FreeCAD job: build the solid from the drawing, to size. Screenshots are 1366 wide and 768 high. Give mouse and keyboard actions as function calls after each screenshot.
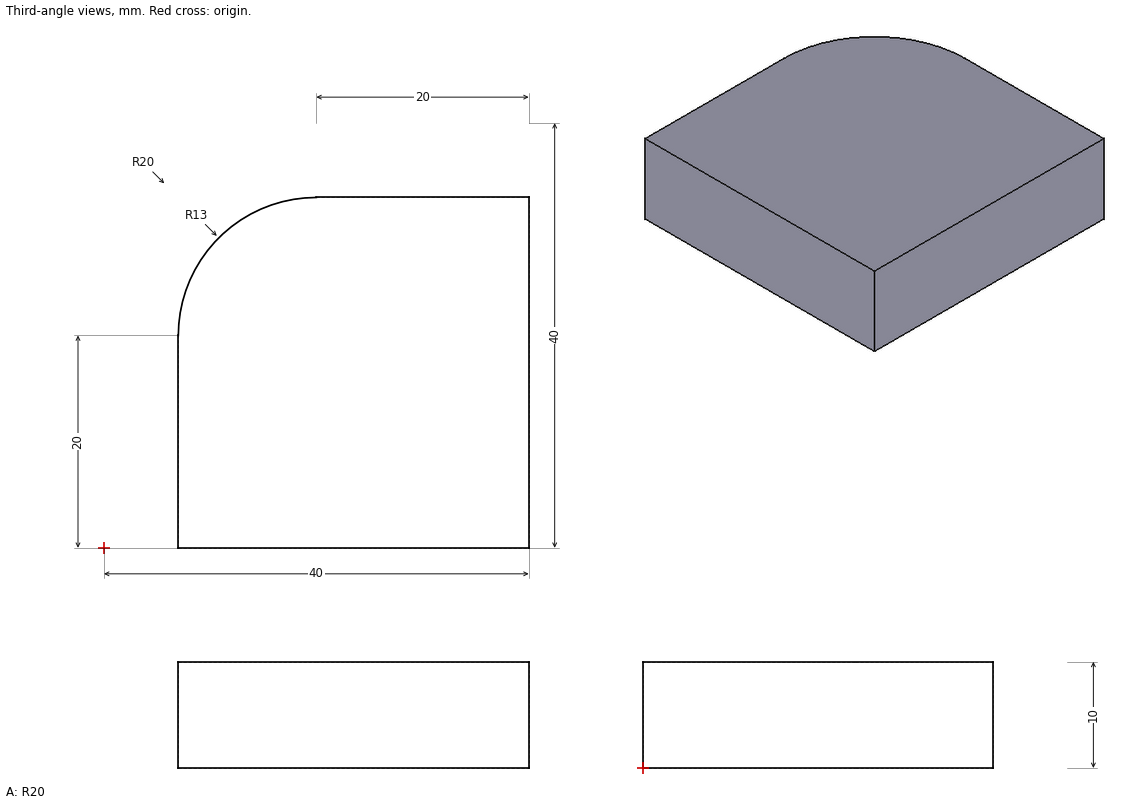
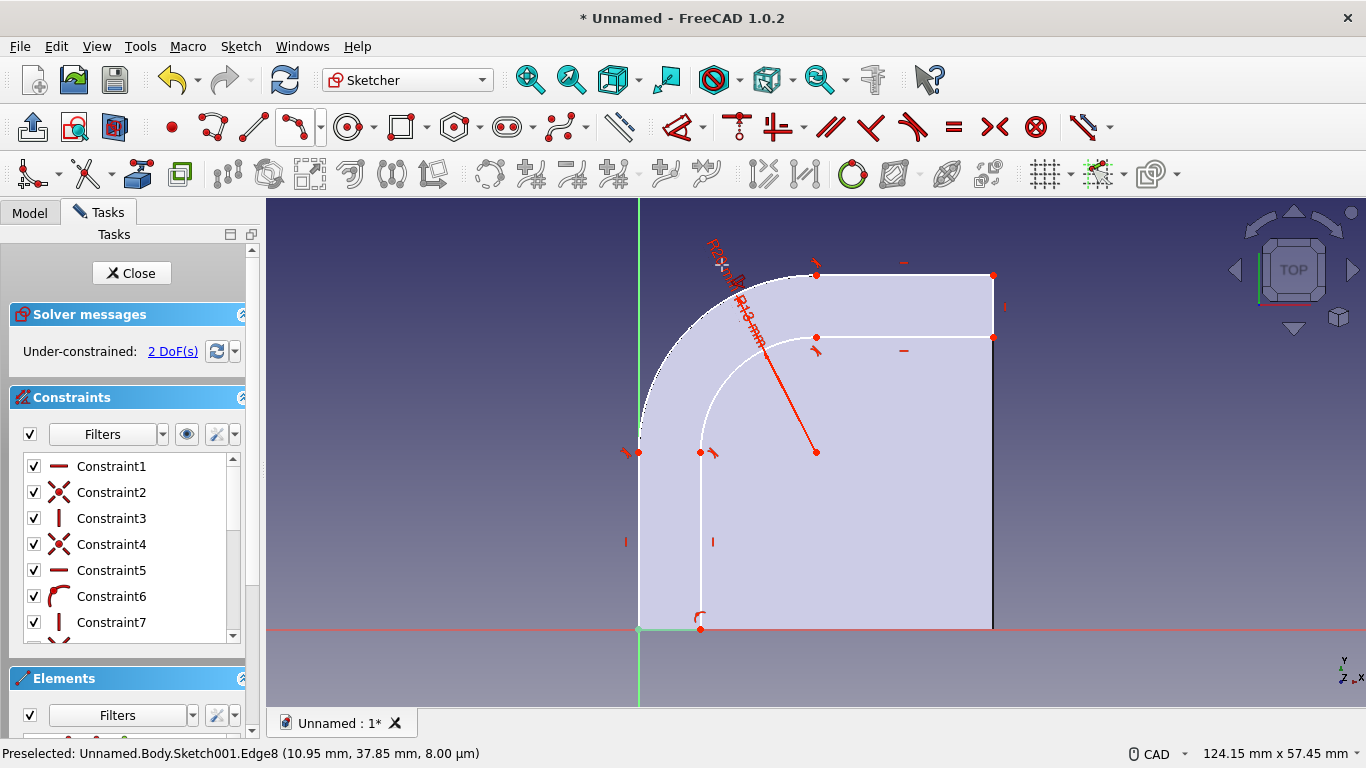
click(869, 275)
click(905, 241)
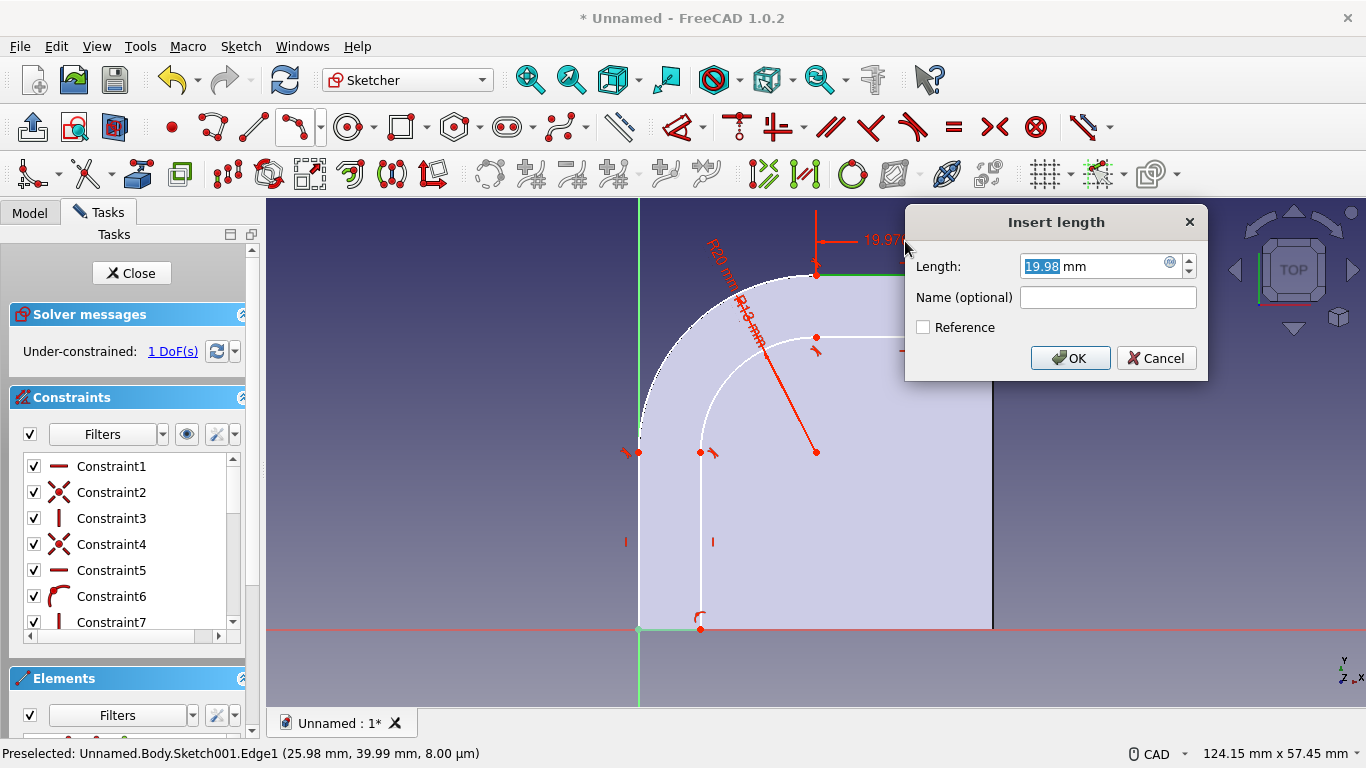
text(20)
key(Return)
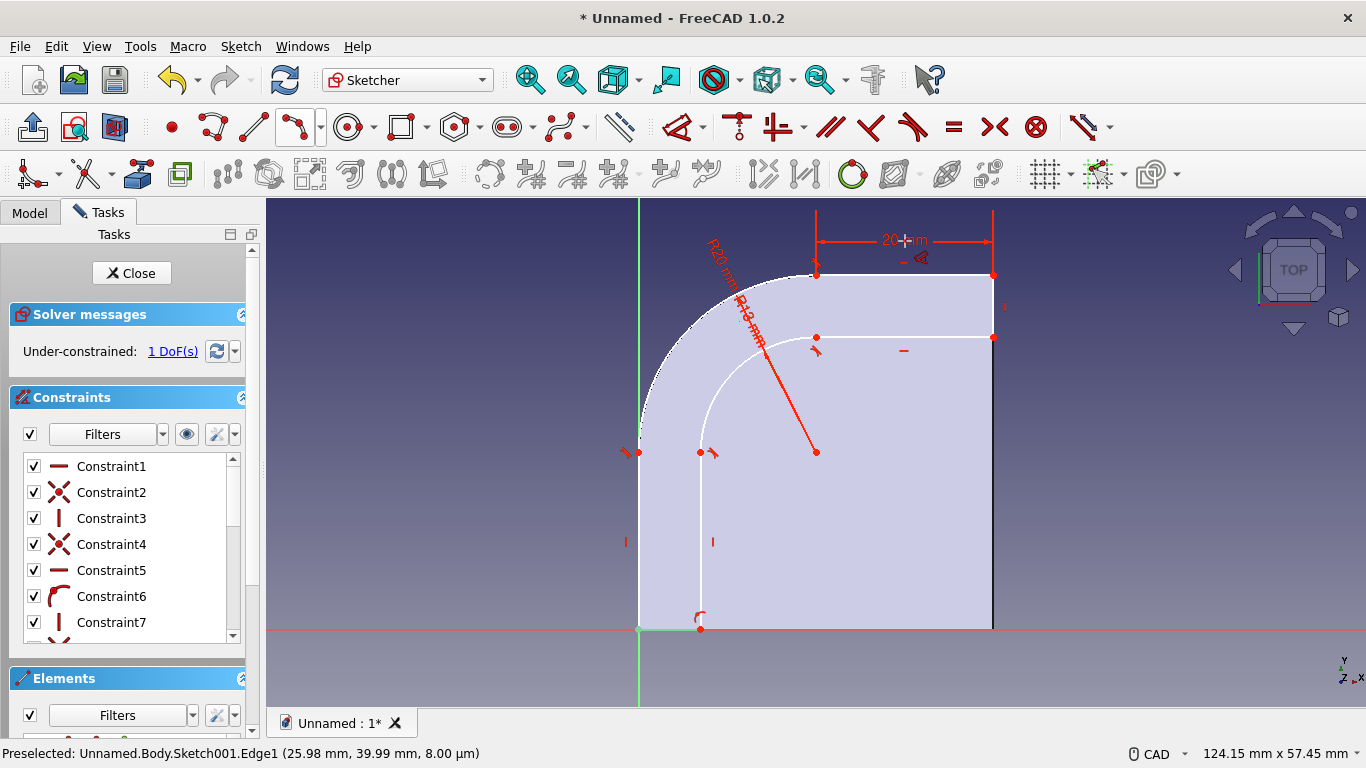
click(701, 506)
click(667, 541)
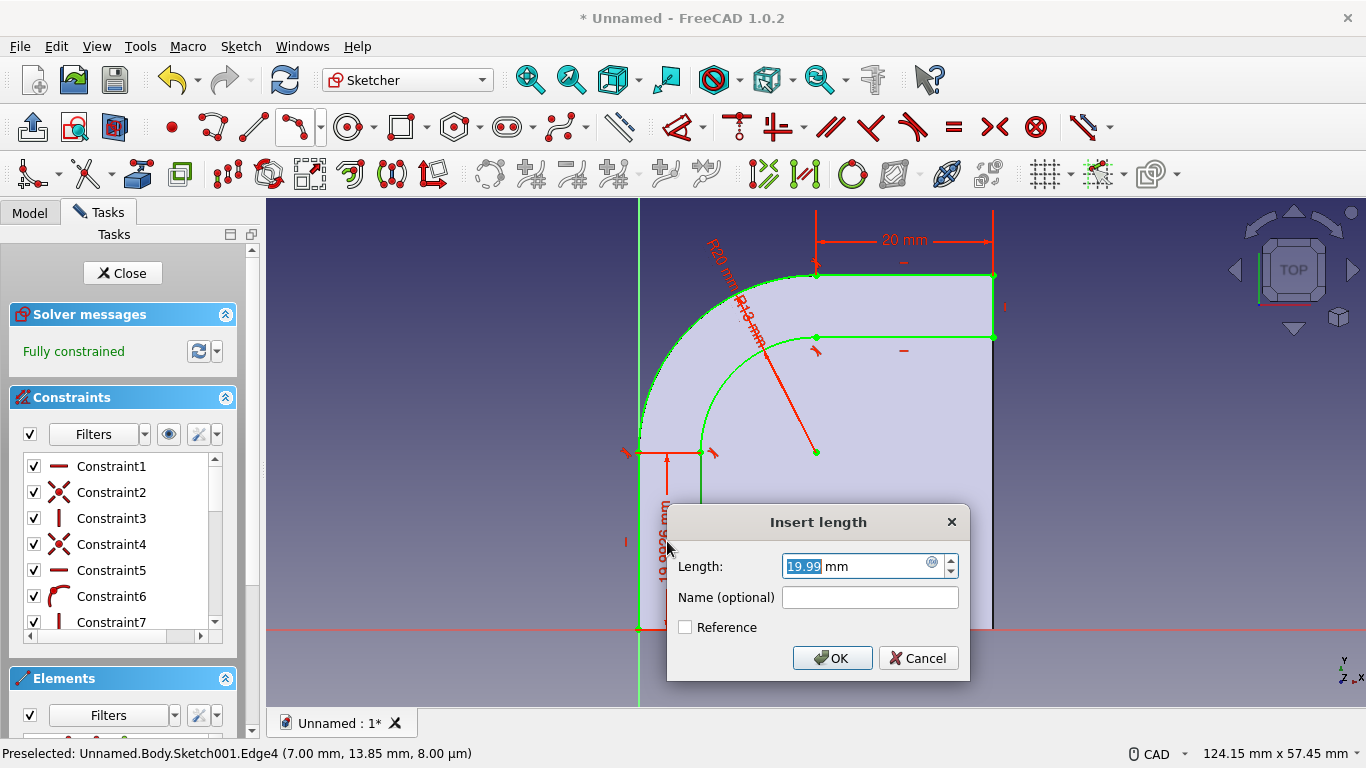
text(20)
key(Return)
key(Escape)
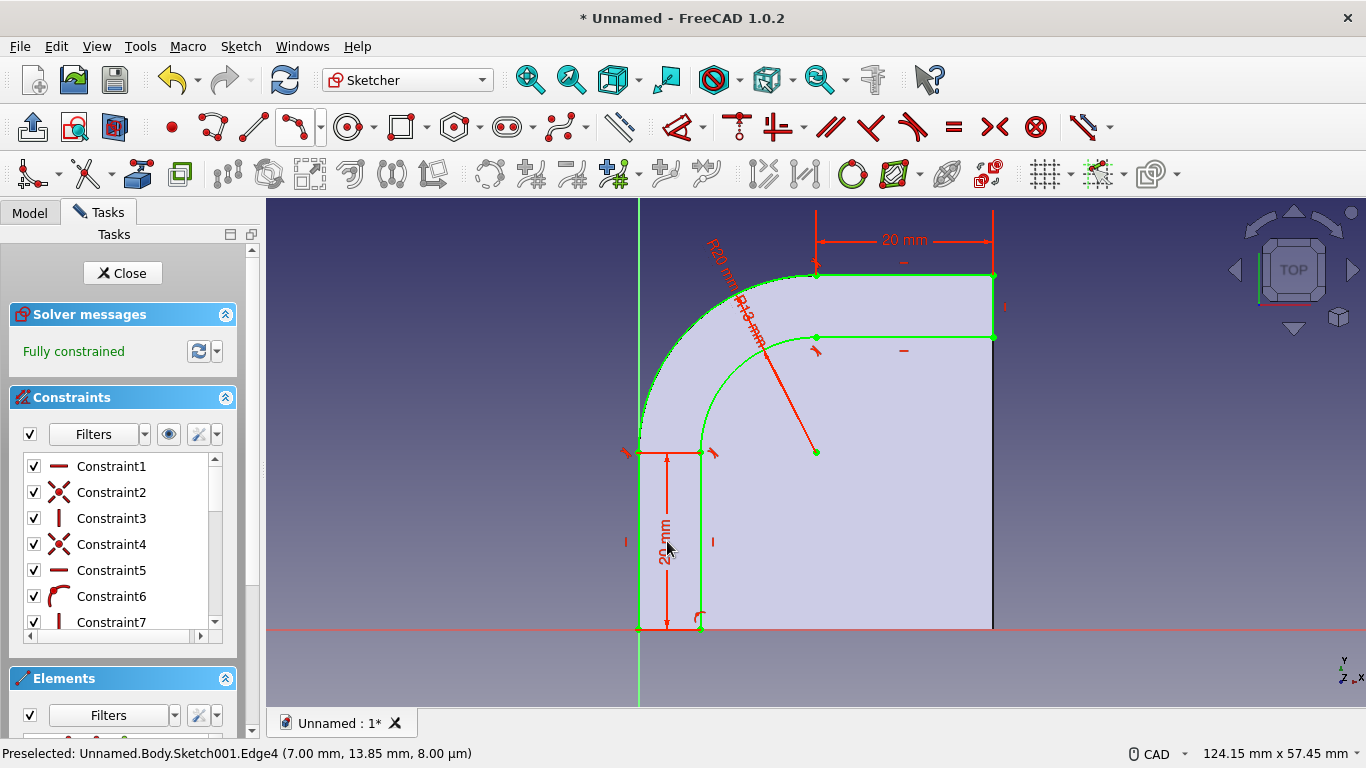
click(123, 273)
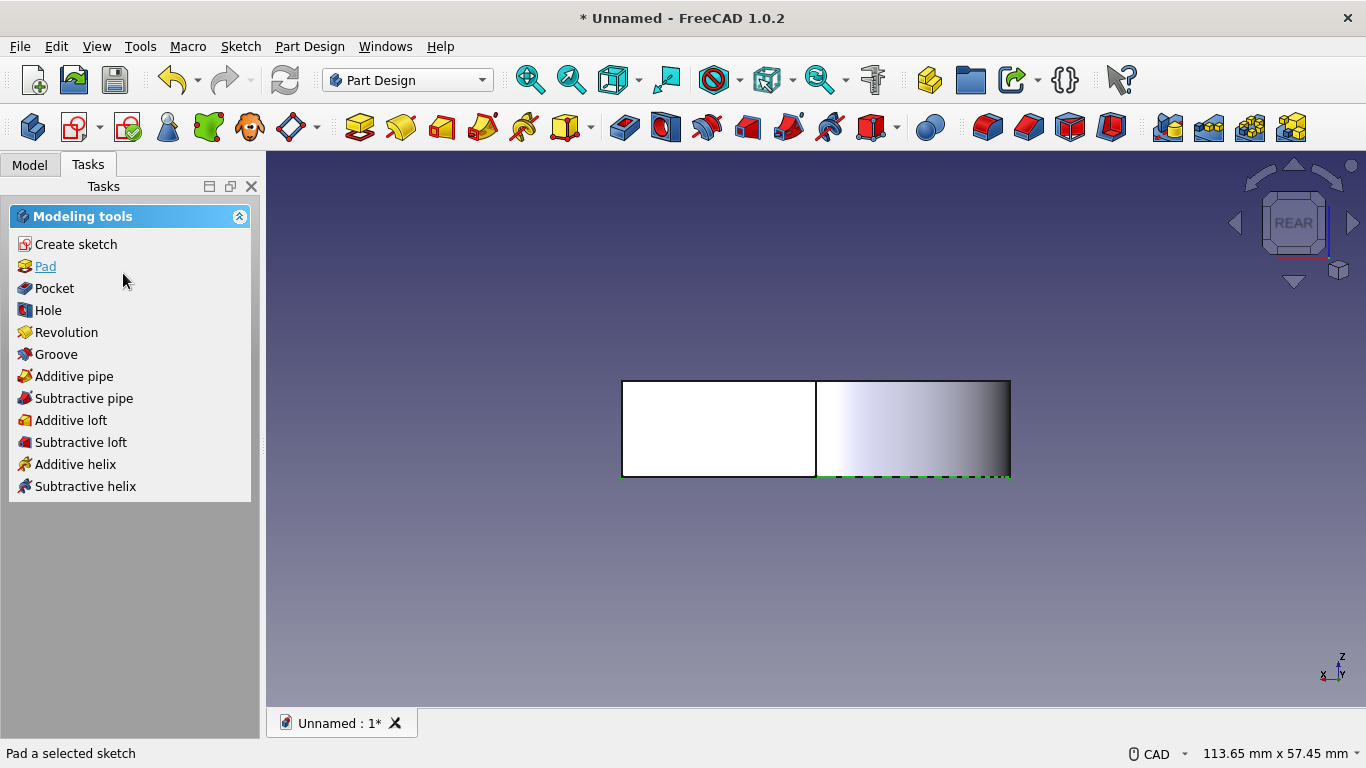
click(625, 128)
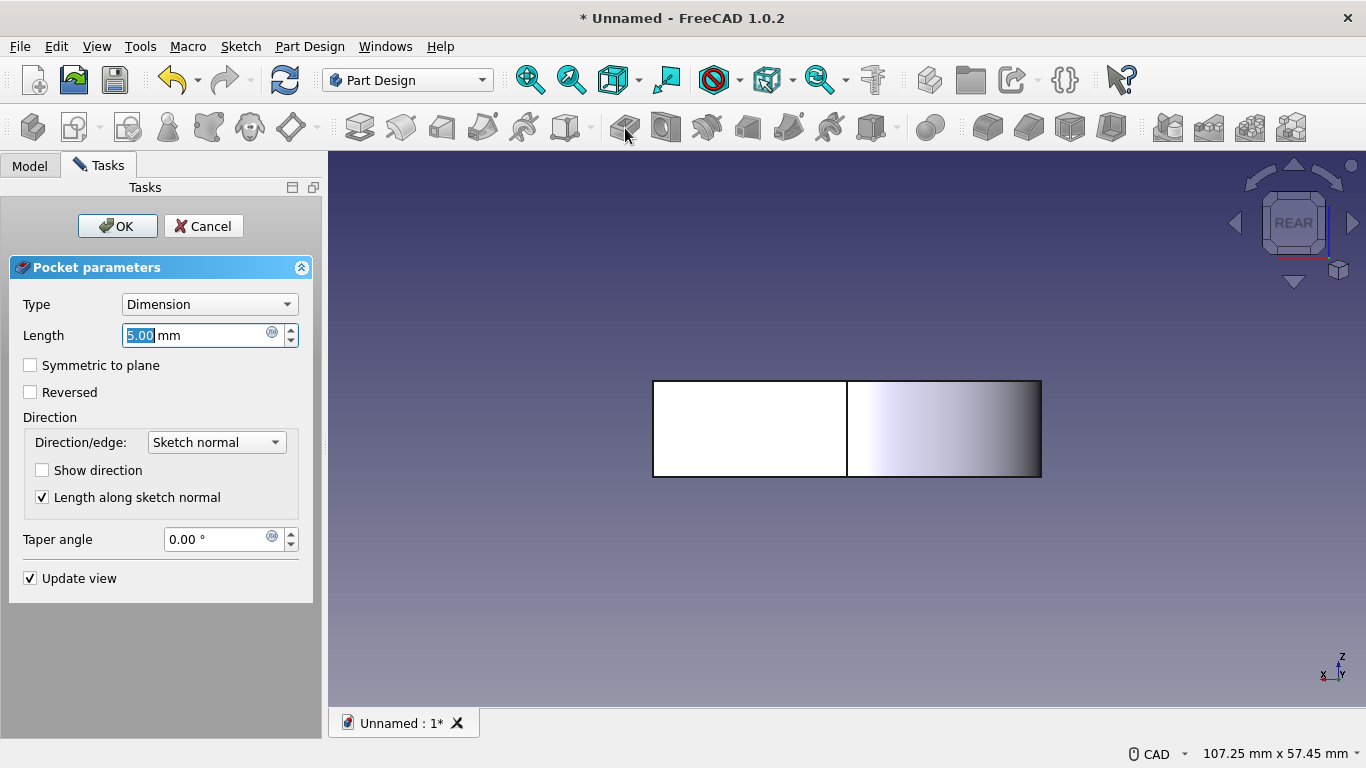
click(210, 304)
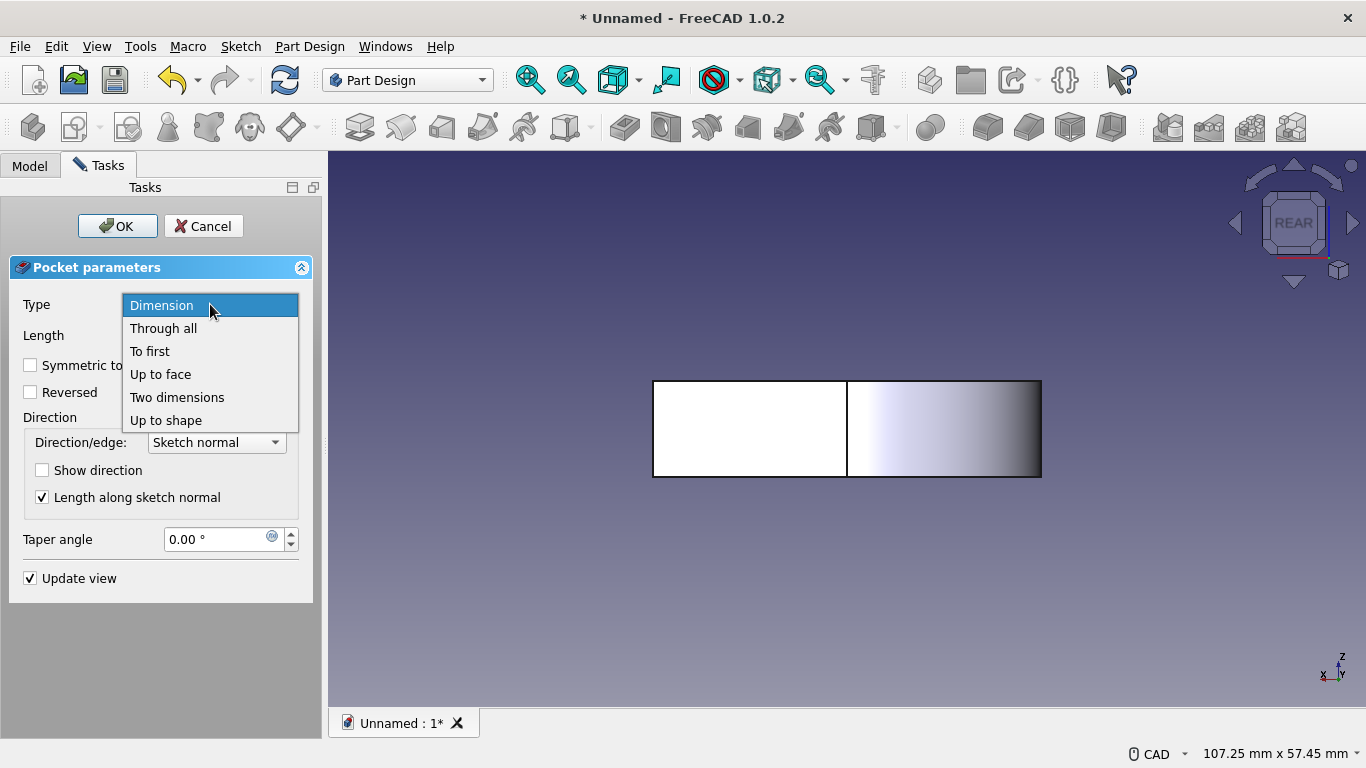
click(208, 328)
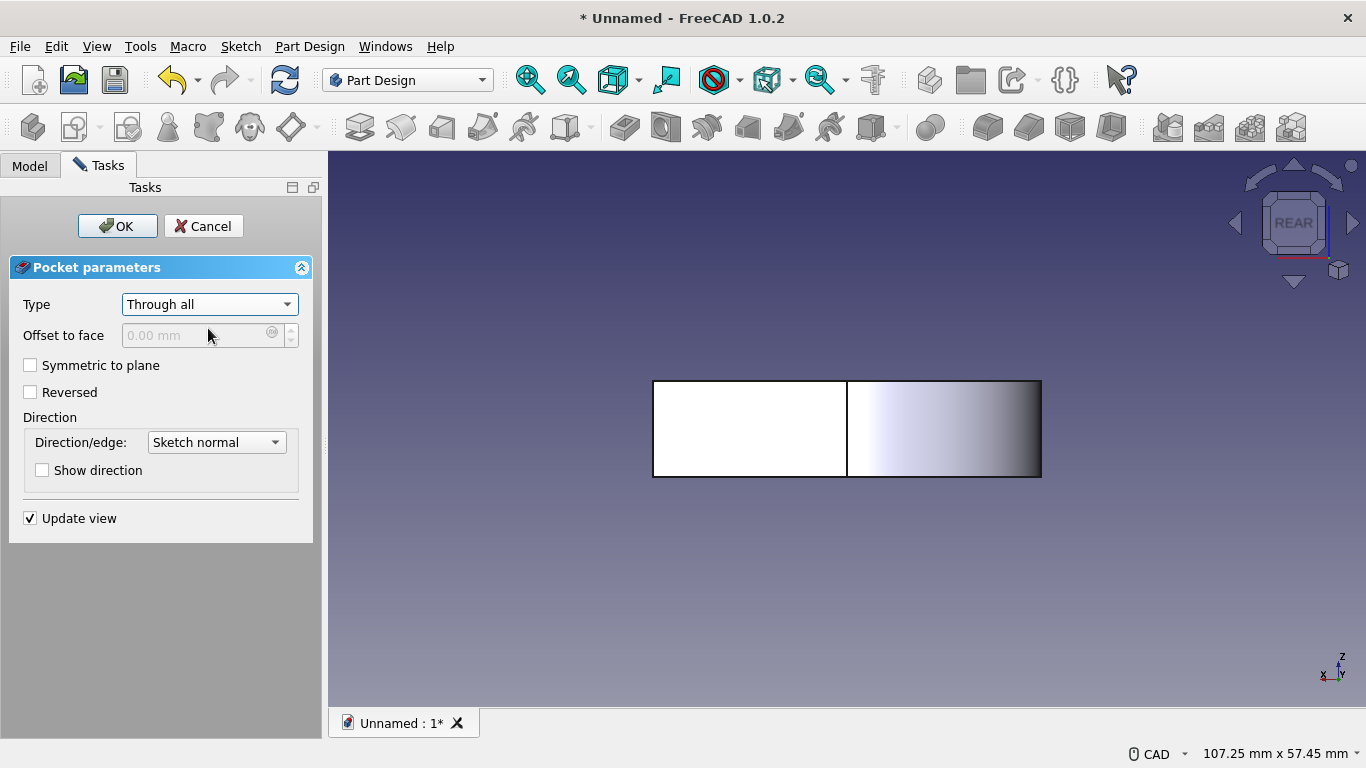
click(31, 392)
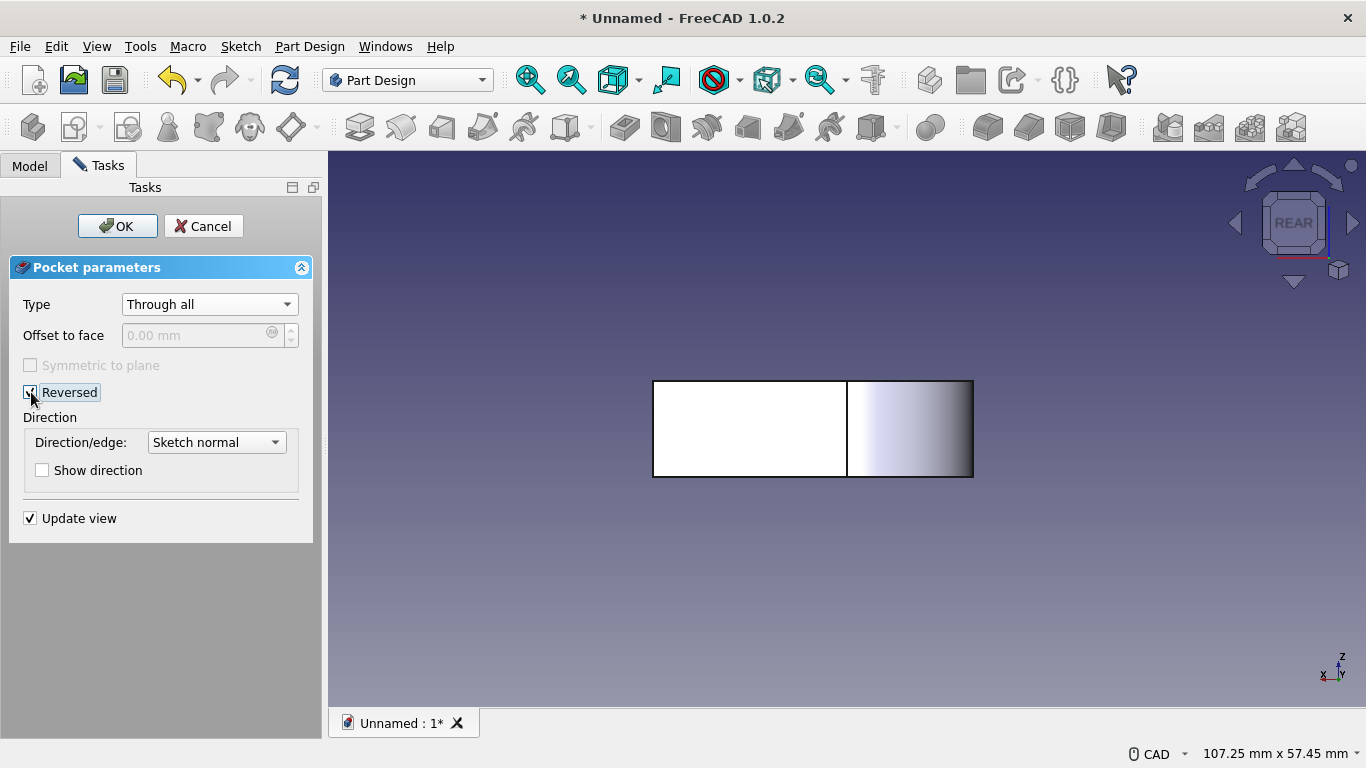
click(118, 226)